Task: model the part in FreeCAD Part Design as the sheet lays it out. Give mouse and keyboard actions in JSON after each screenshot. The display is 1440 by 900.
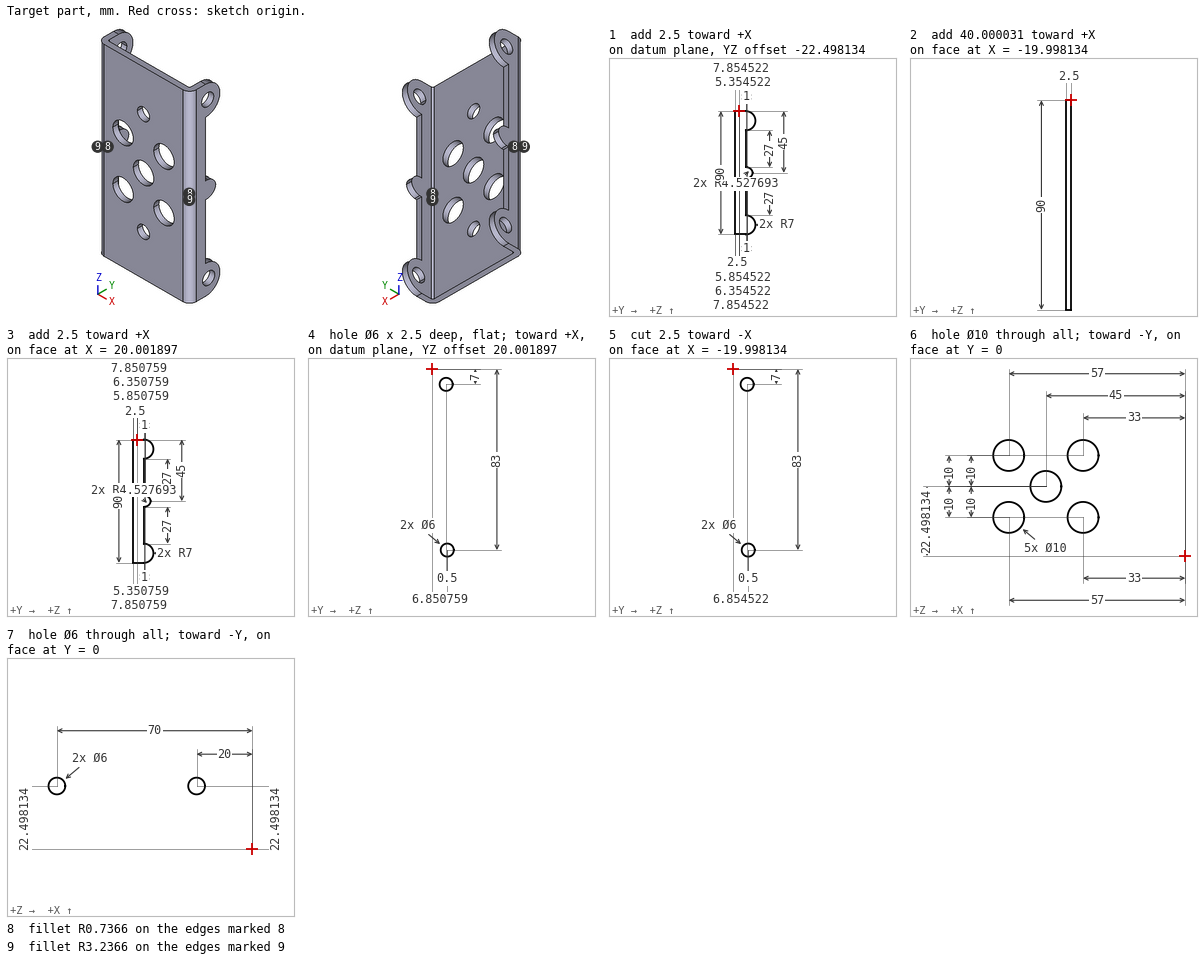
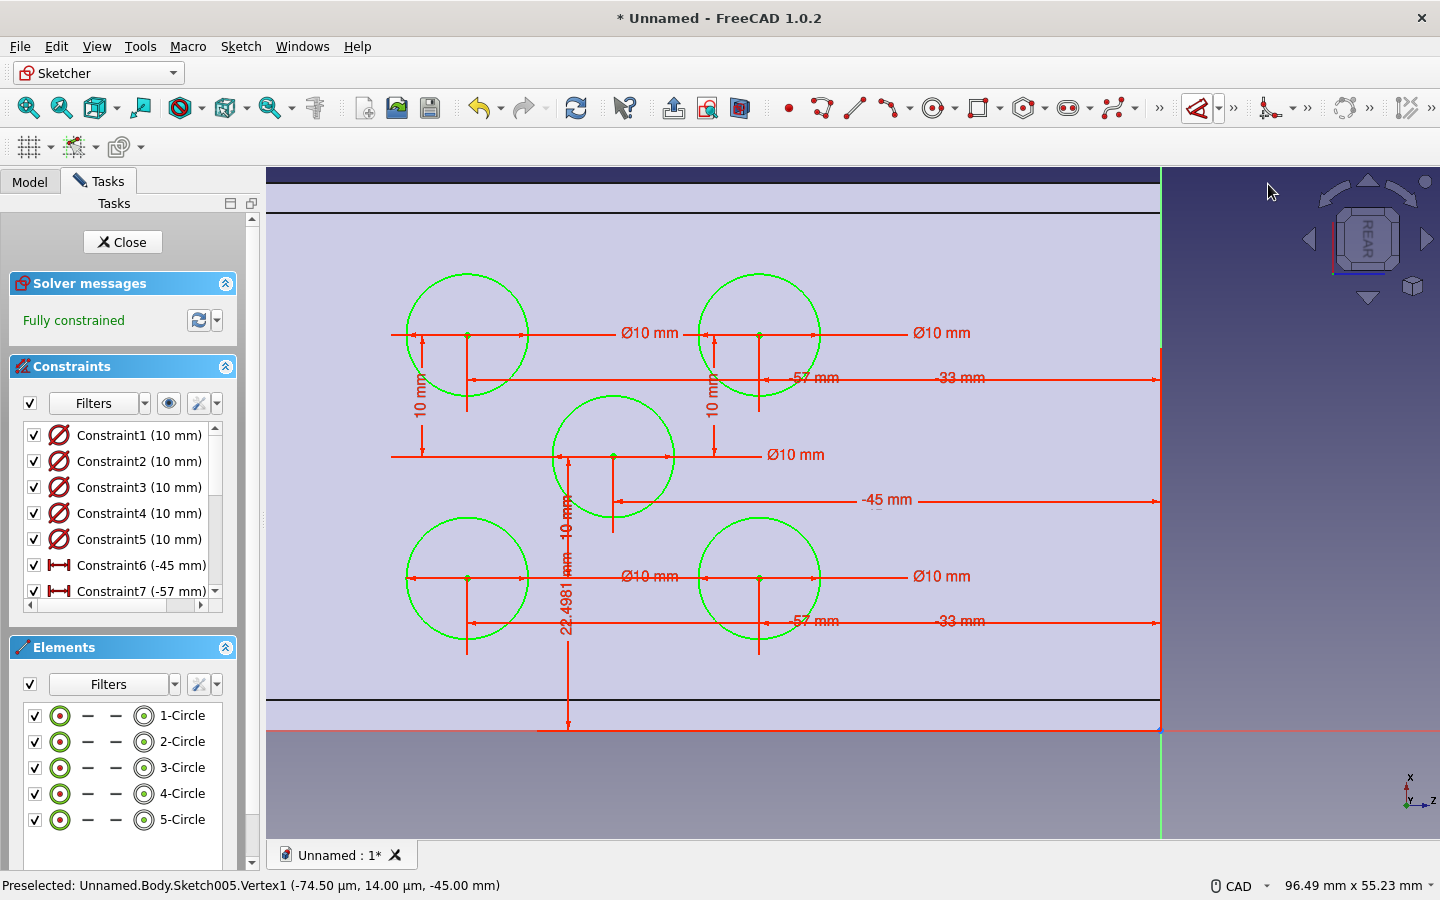
{"action": "left_click", "coordinate": [123, 242]}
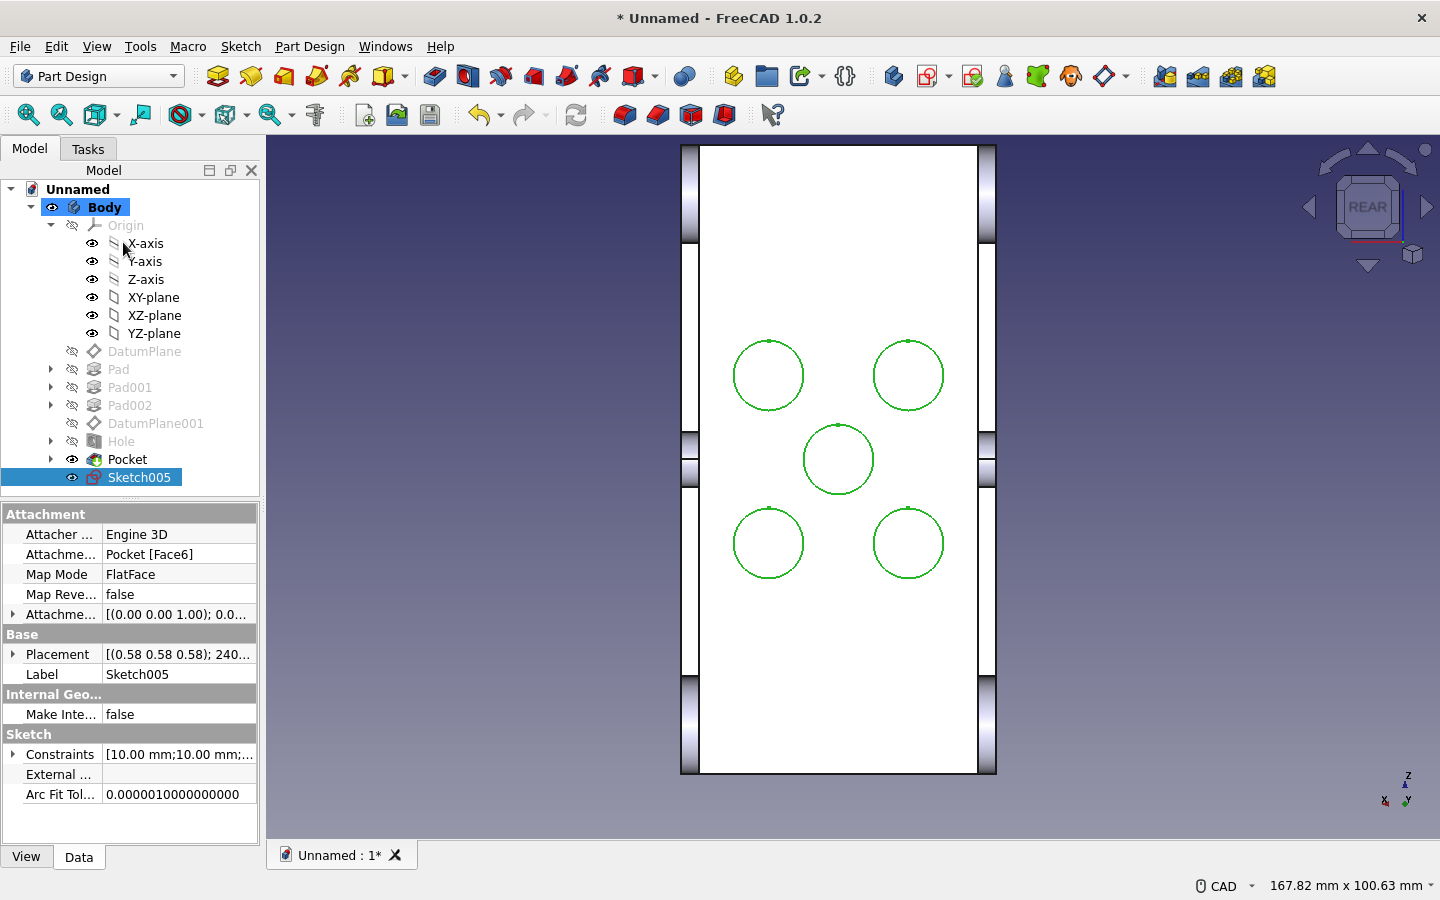
{"action": "left_click", "coordinate": [468, 76]}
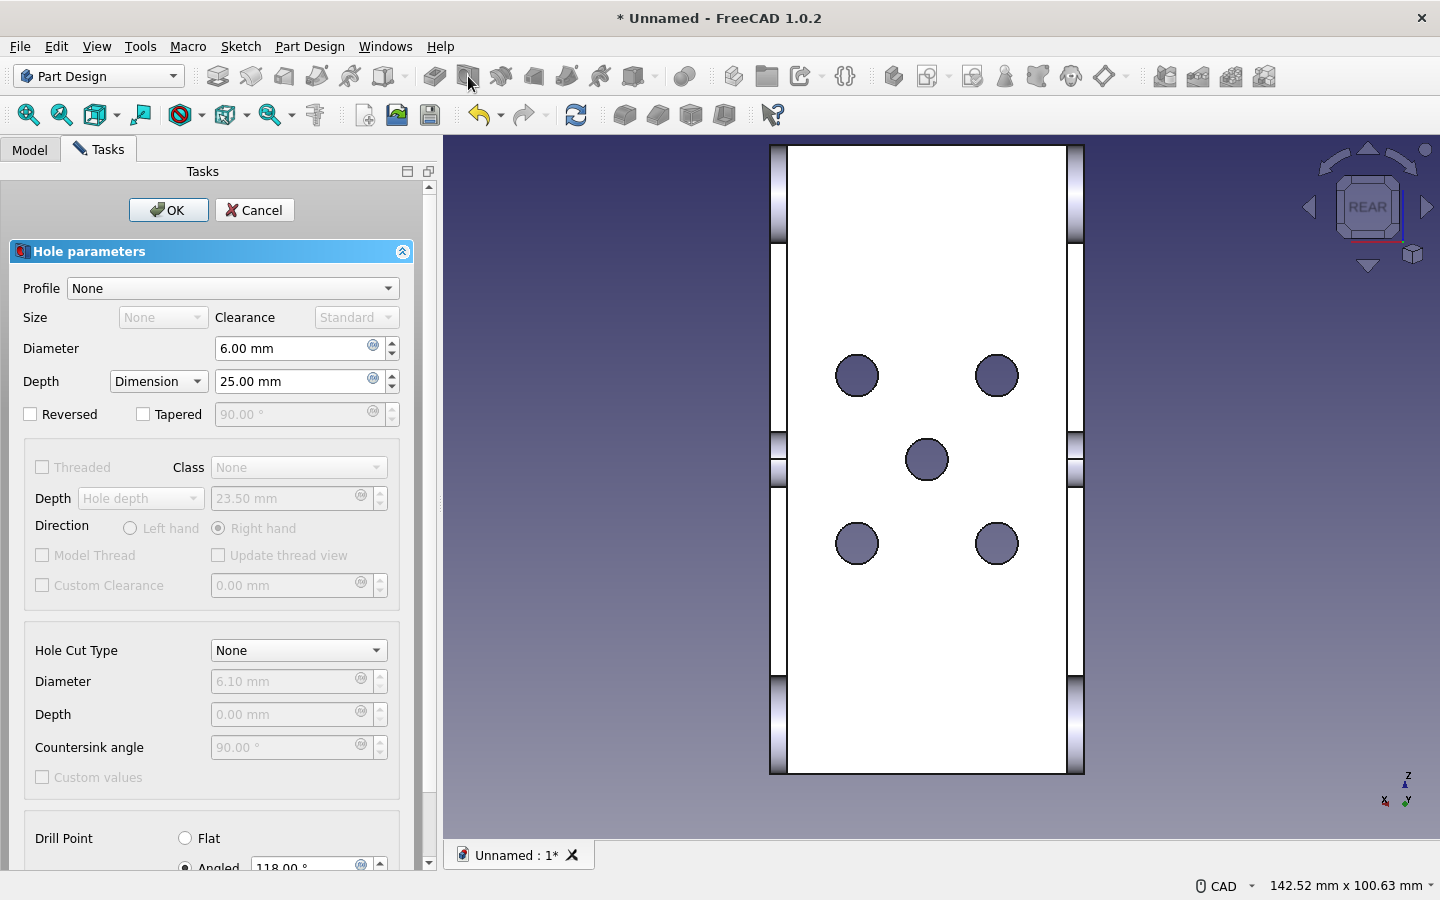
{"action": "triple_click", "coordinate": [300, 348]}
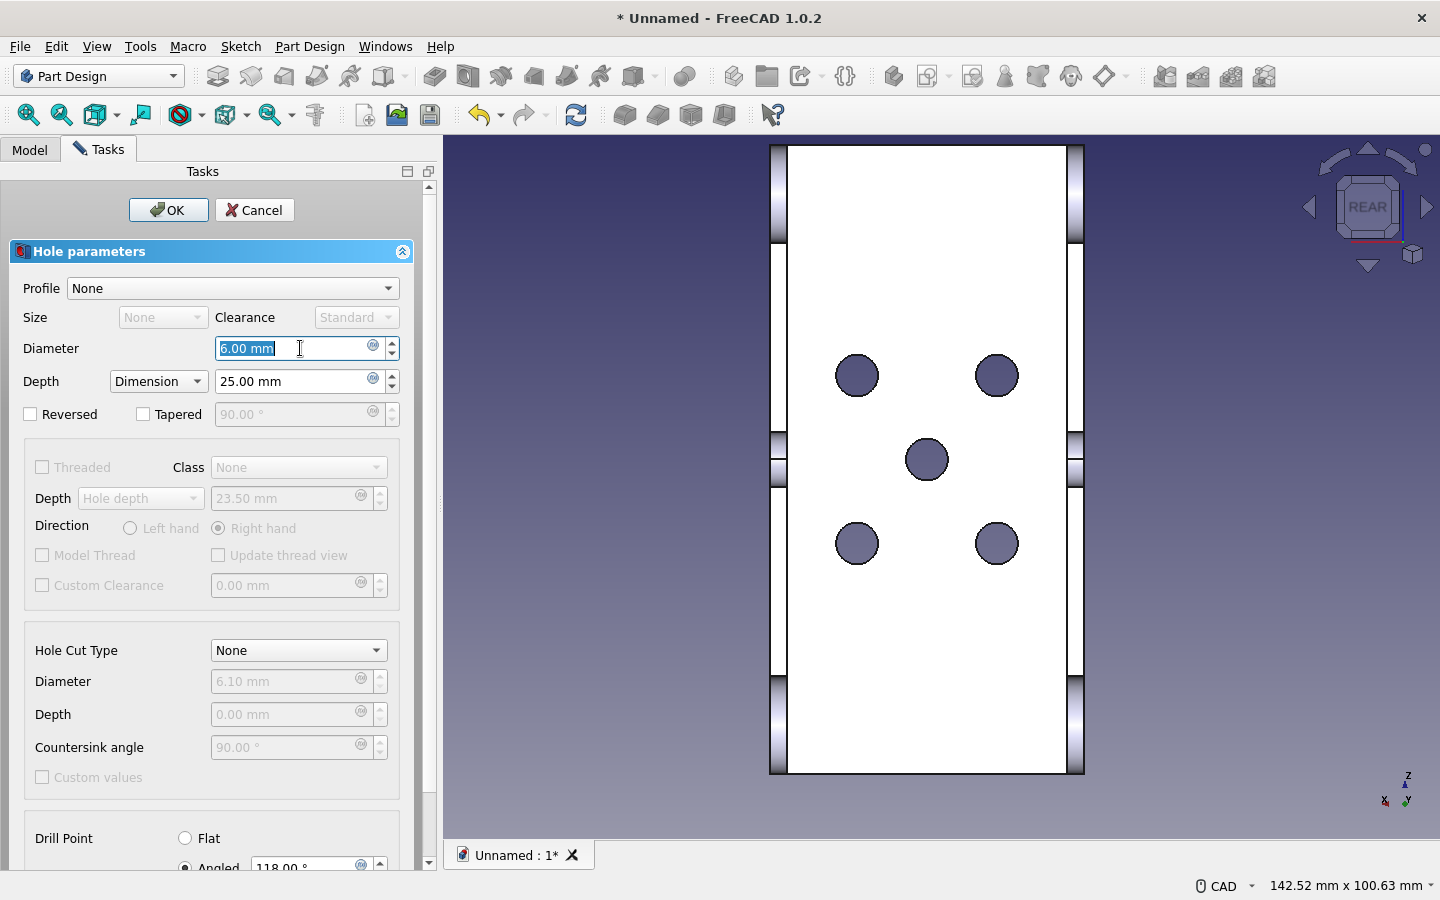
{"action": "type", "text": "10"}
{"action": "key", "text": "Tab"}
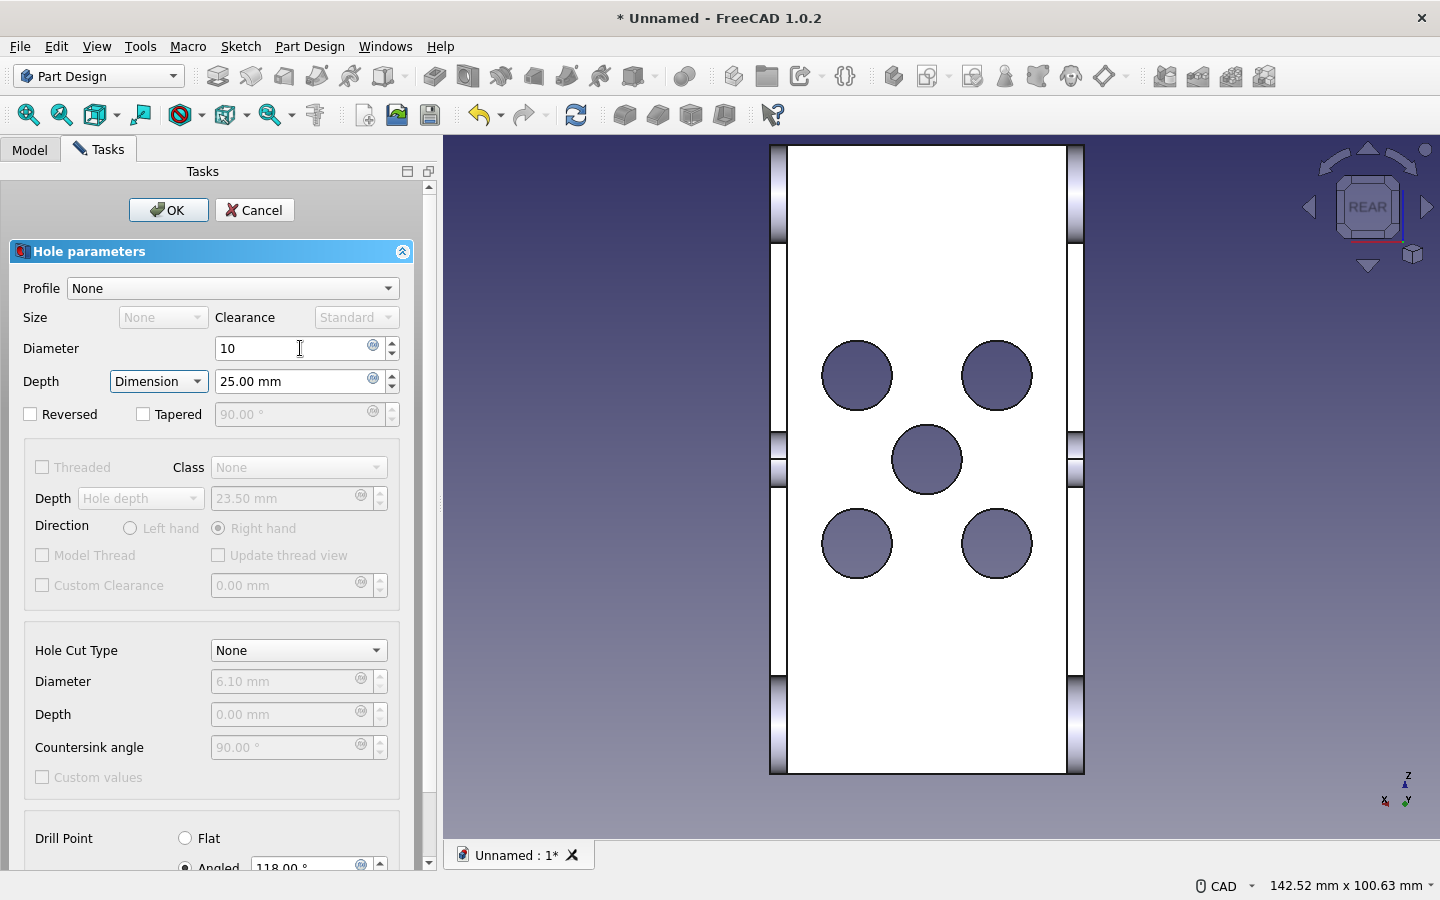
{"action": "left_click", "coordinate": [160, 382]}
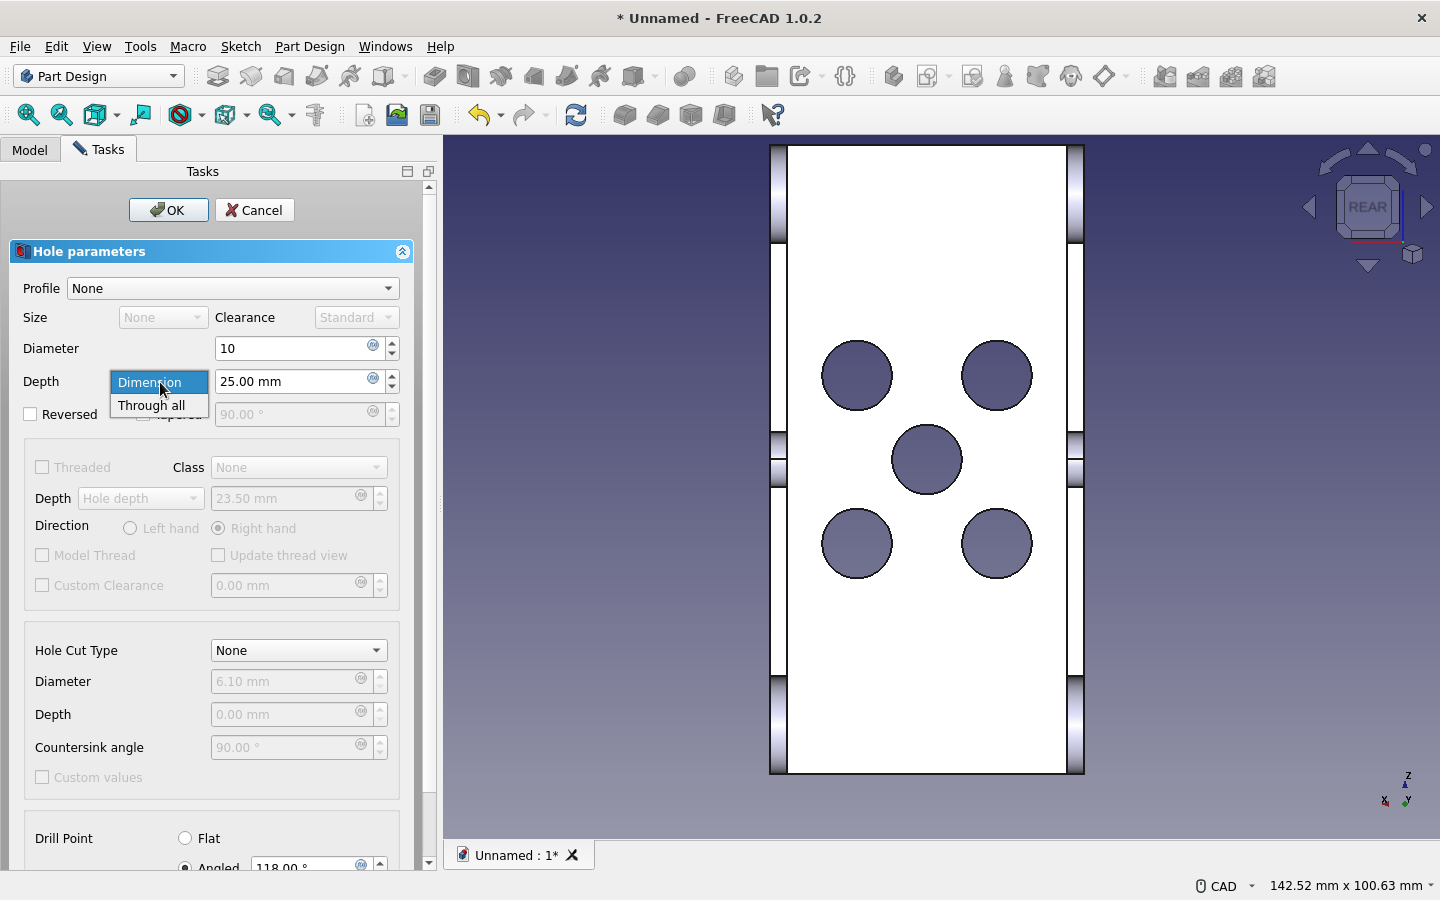
{"action": "left_click", "coordinate": [158, 406]}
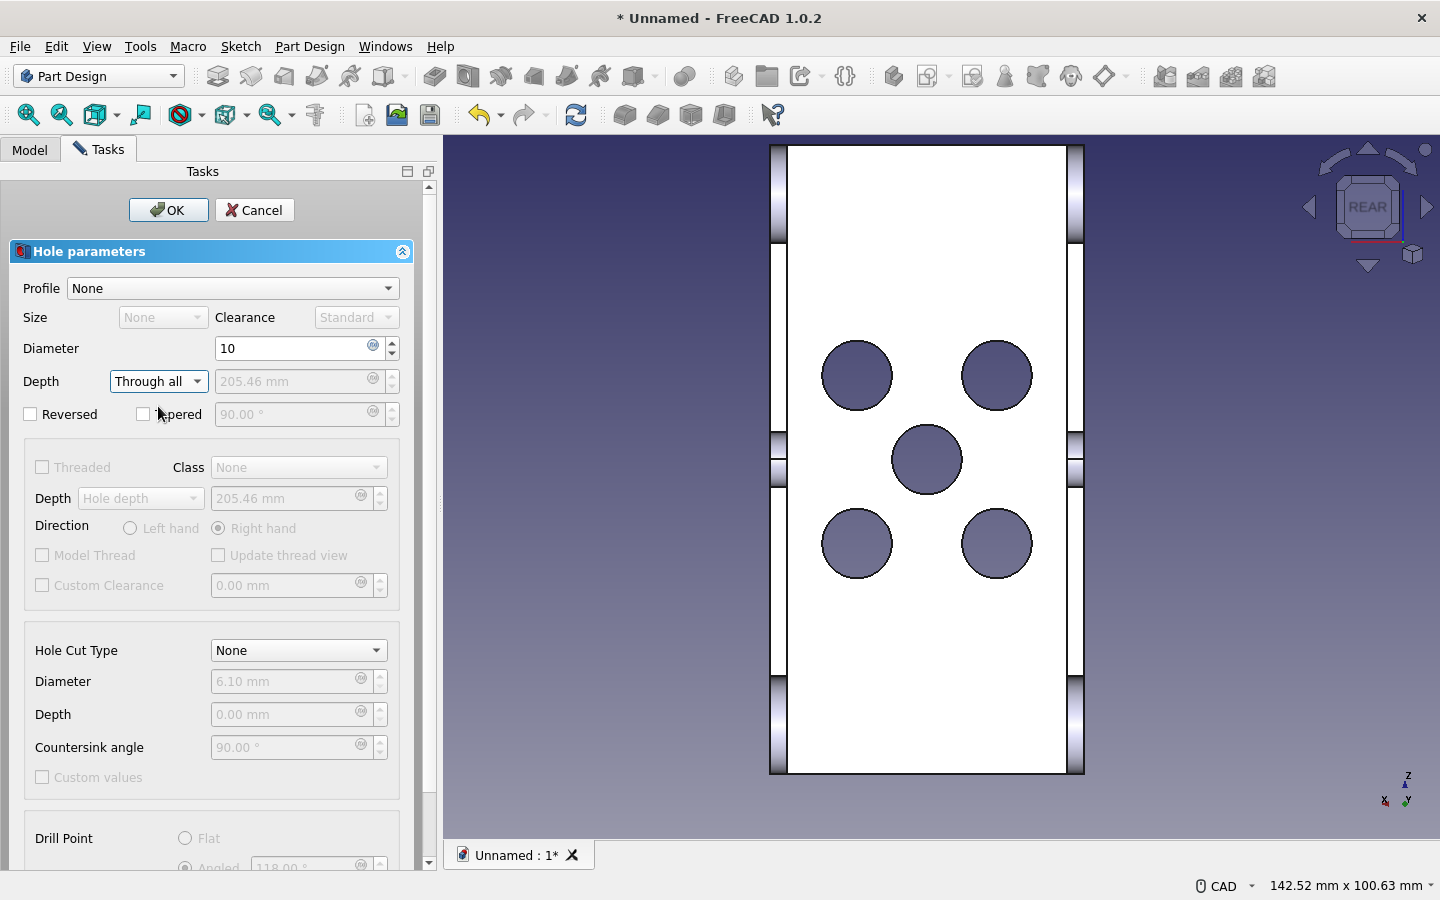
{"action": "left_click", "coordinate": [169, 210]}